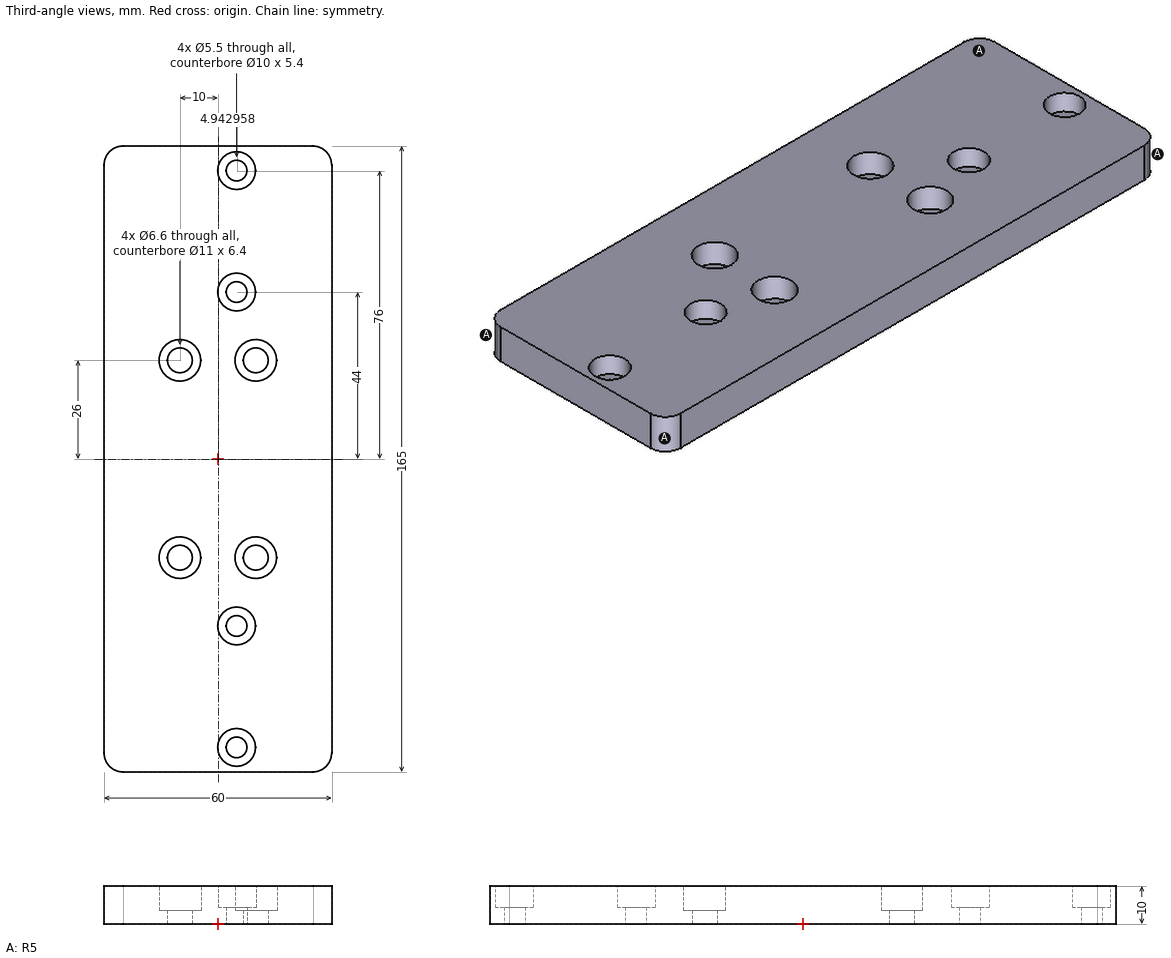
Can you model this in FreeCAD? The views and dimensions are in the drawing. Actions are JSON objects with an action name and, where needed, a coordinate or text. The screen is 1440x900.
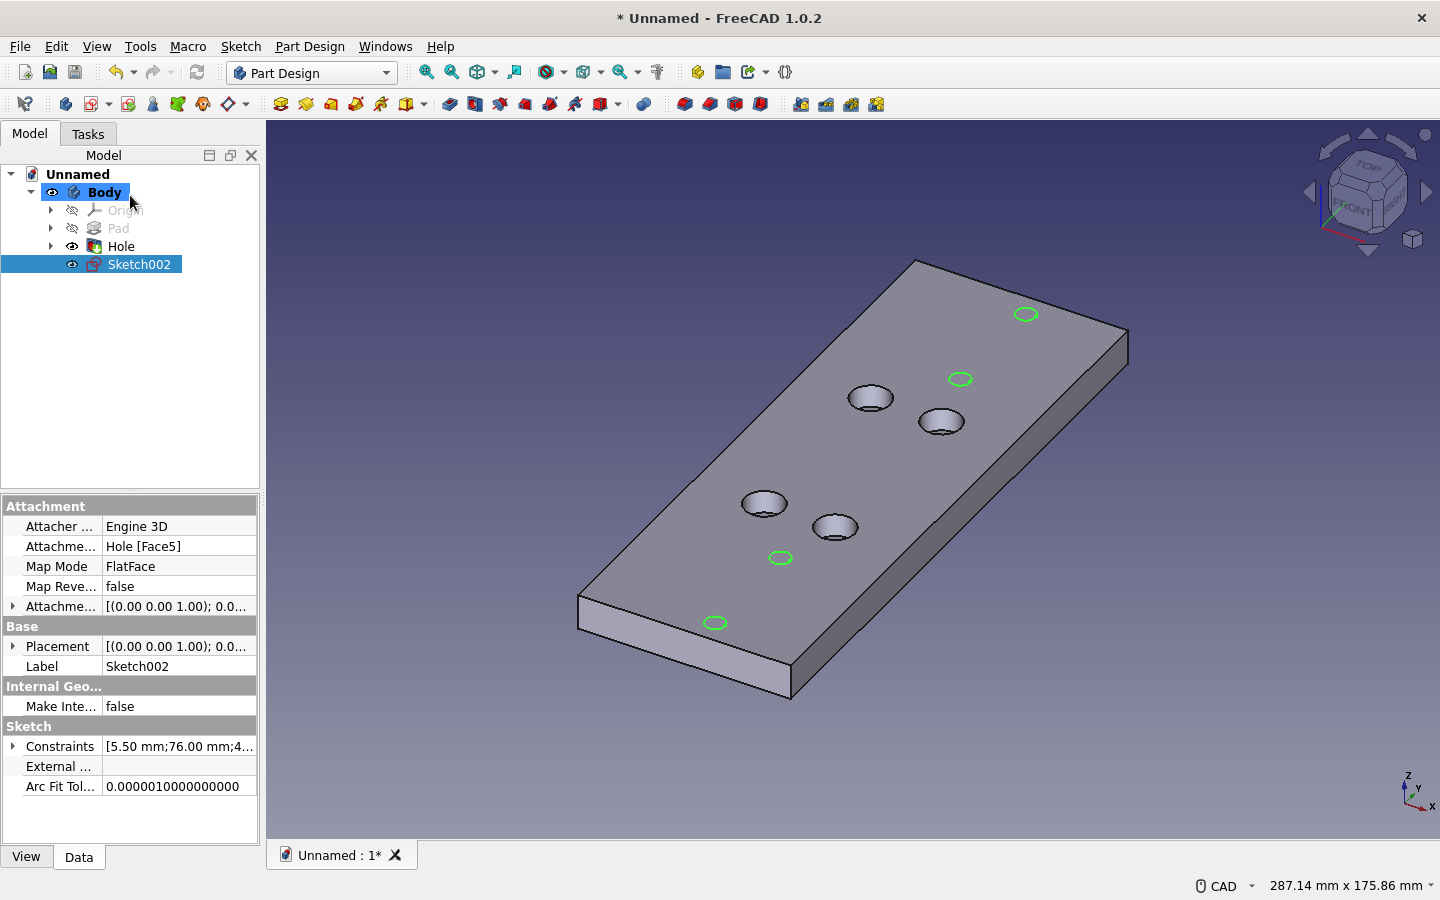
{"action": "left_click", "coordinate": [475, 104]}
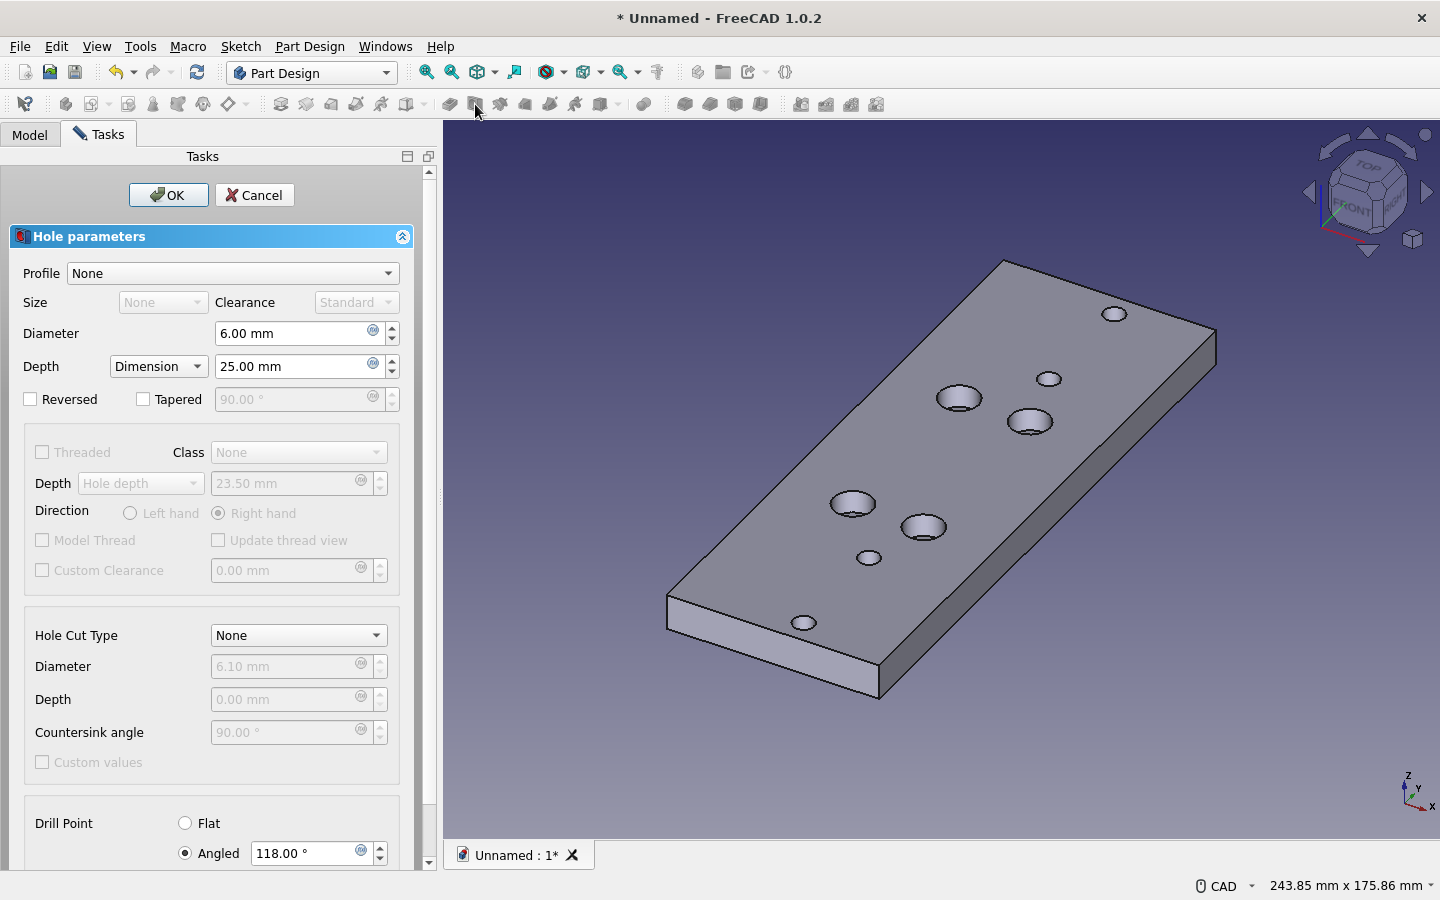
{"action": "triple_click", "coordinate": [300, 334]}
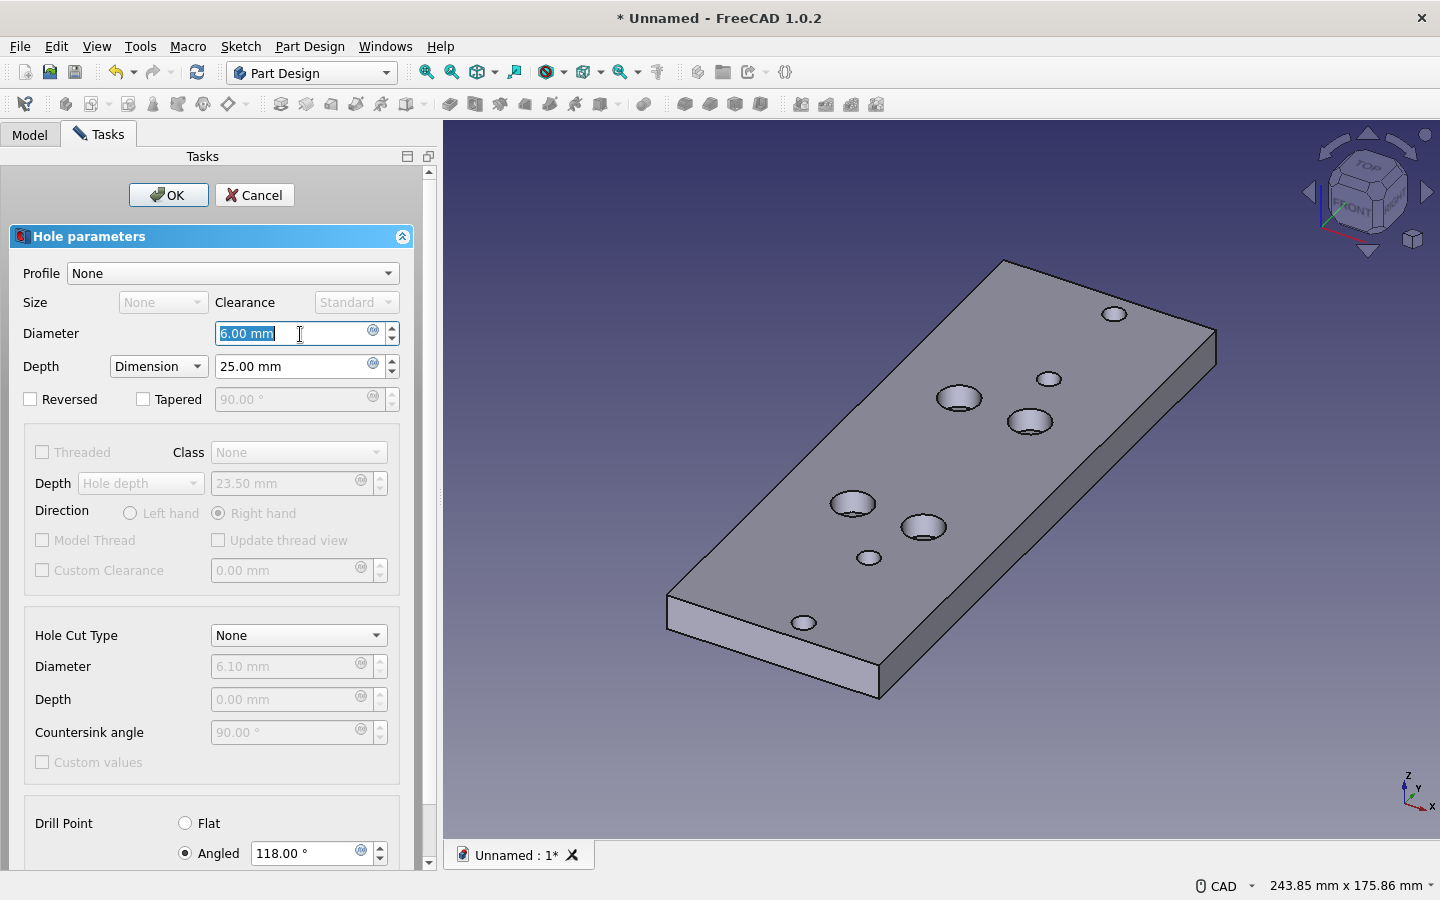
{"action": "type", "text": "5.5"}
{"action": "key", "text": "Tab"}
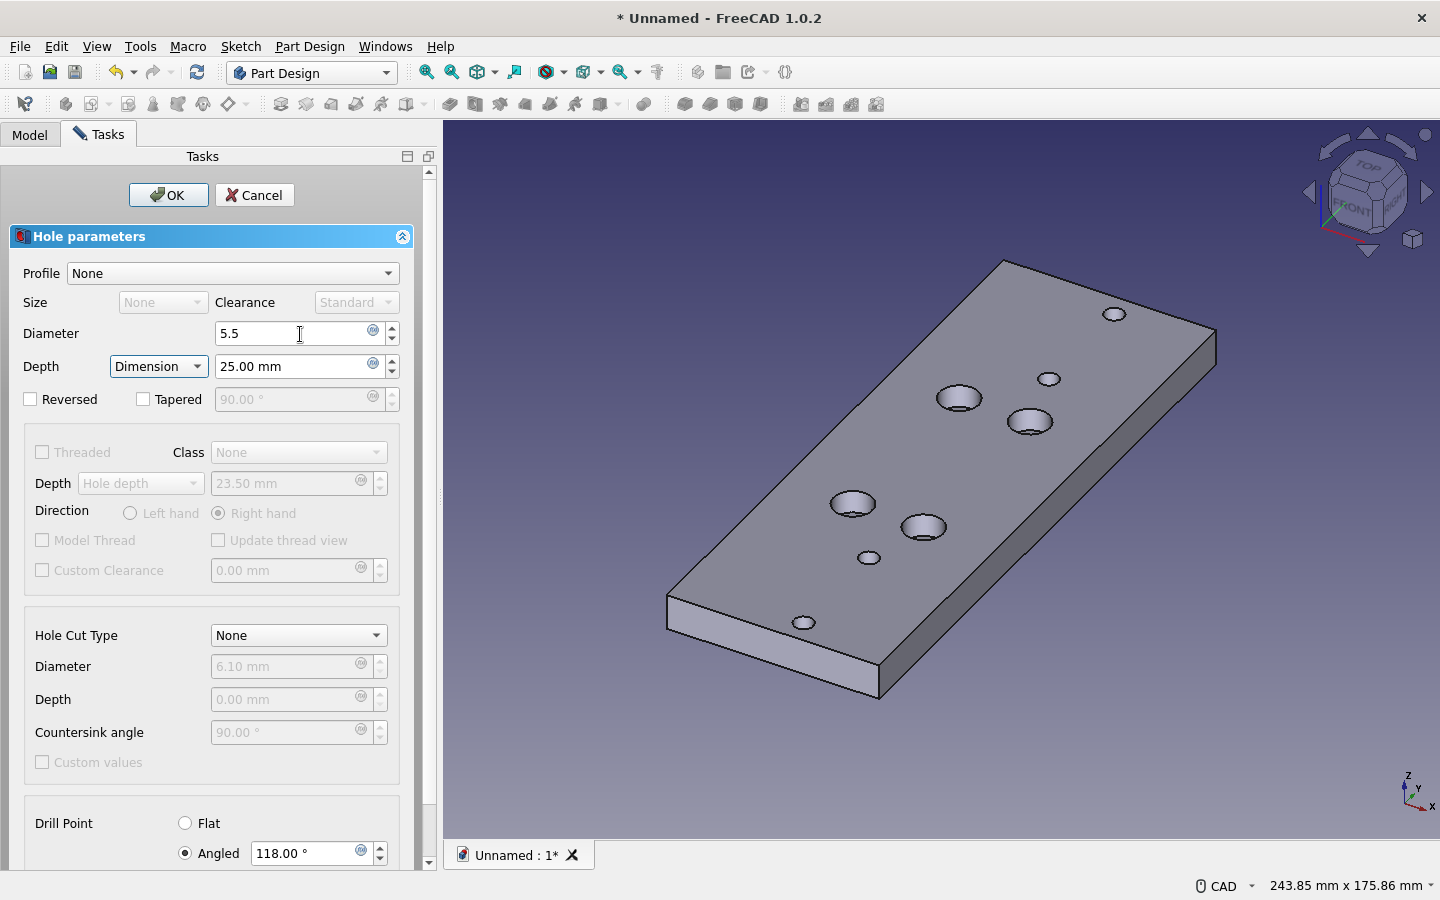
{"action": "left_click", "coordinate": [160, 366]}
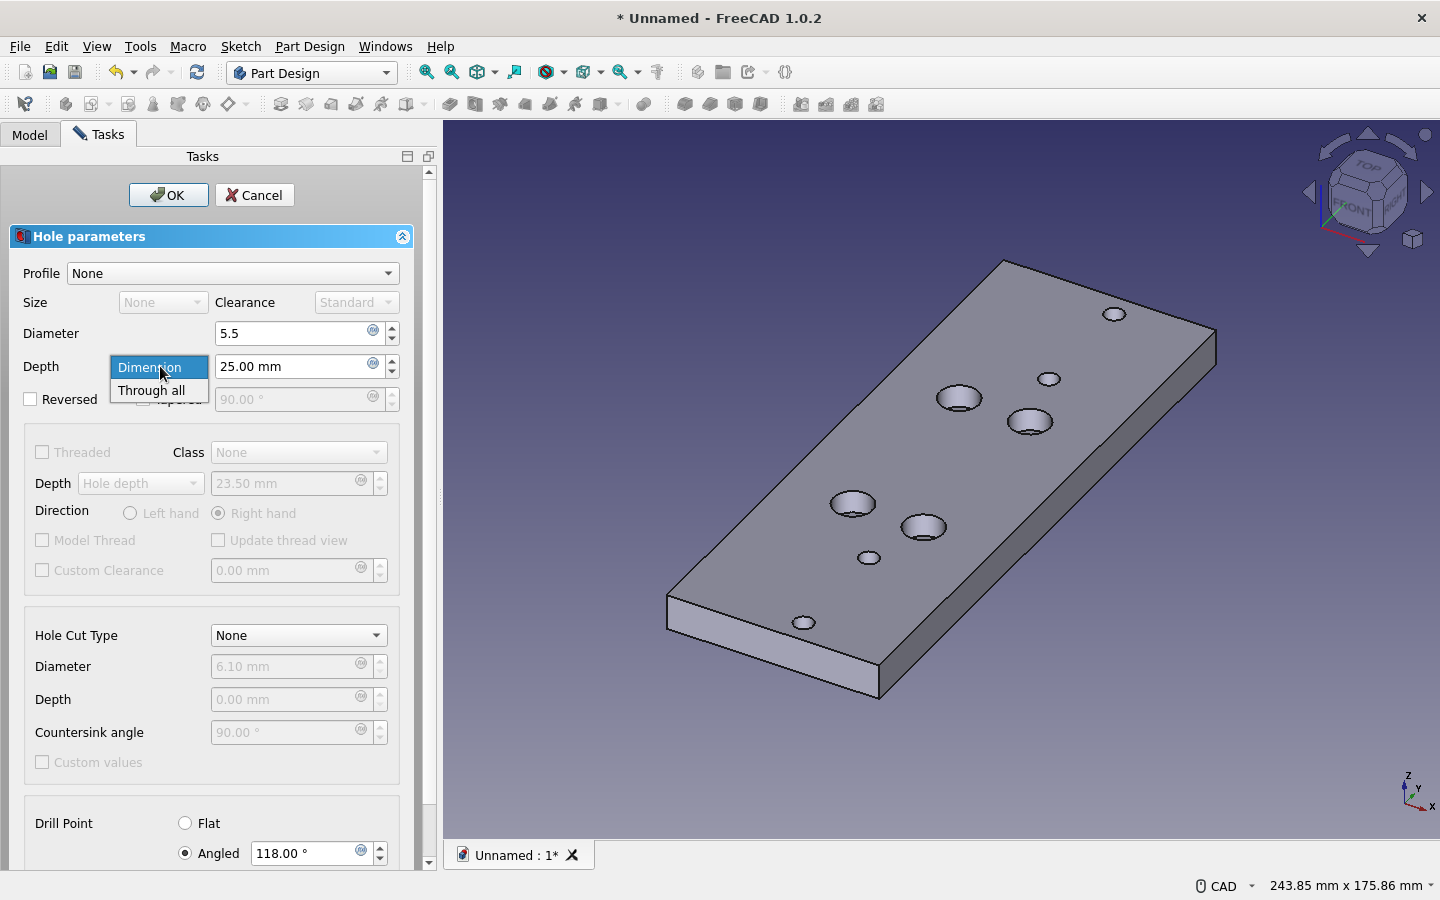
{"action": "left_click", "coordinate": [158, 390]}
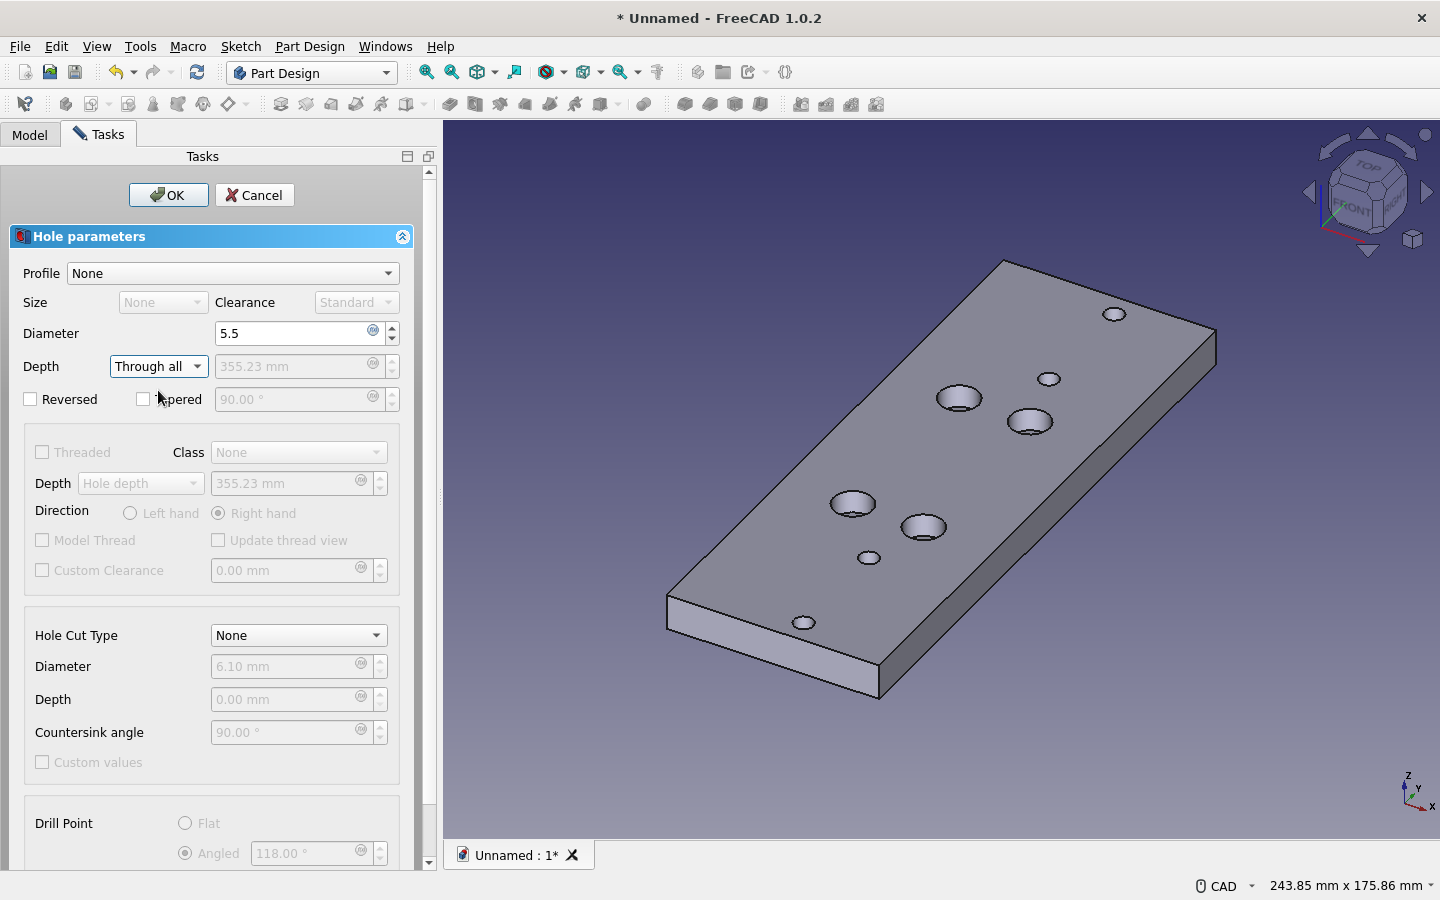
{"action": "left_click", "coordinate": [300, 636]}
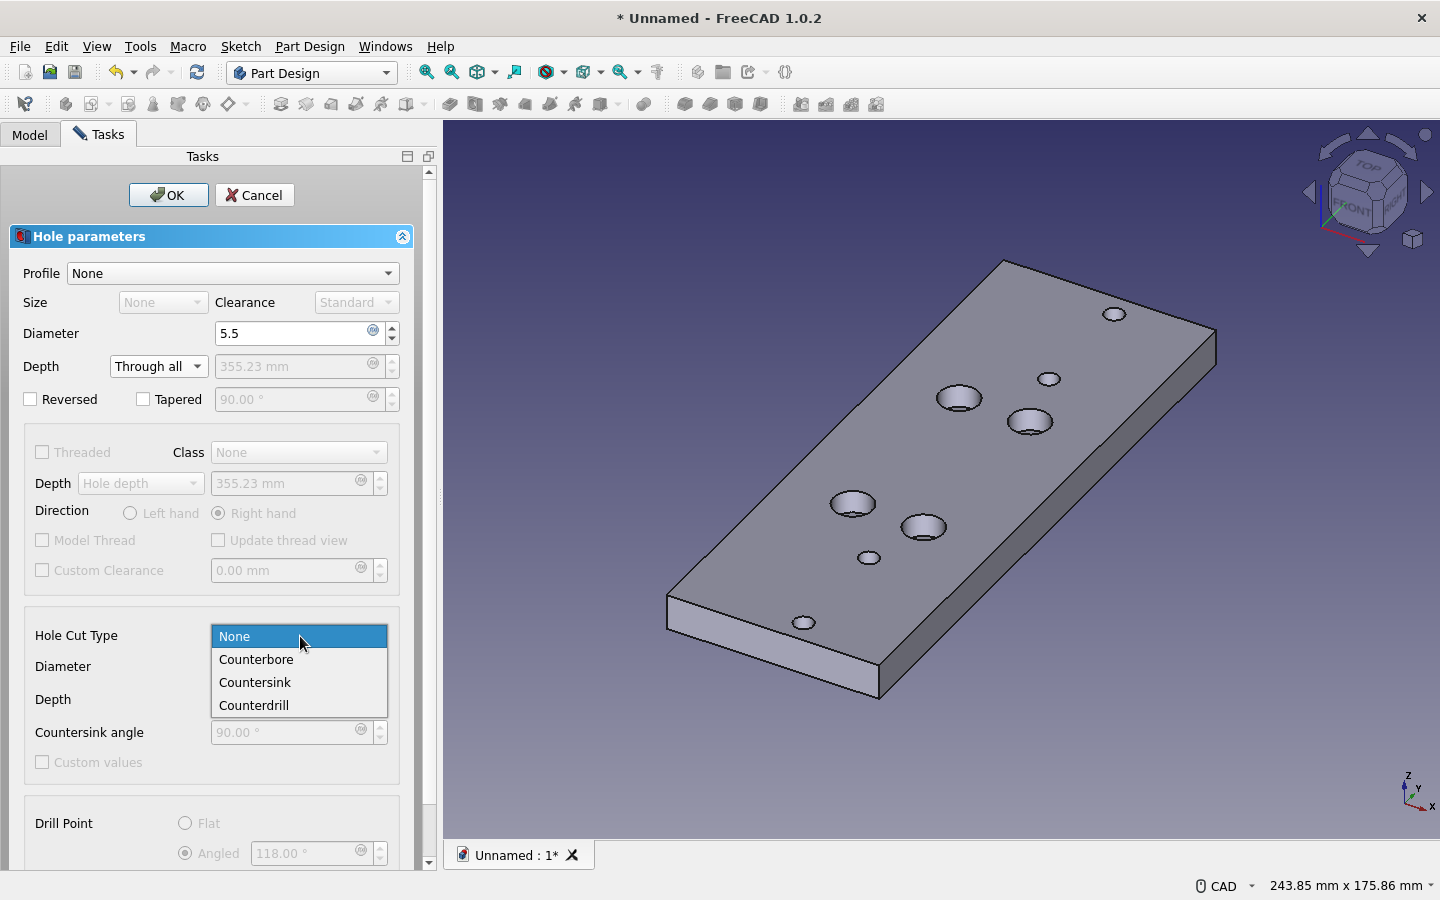
{"action": "left_click", "coordinate": [298, 660]}